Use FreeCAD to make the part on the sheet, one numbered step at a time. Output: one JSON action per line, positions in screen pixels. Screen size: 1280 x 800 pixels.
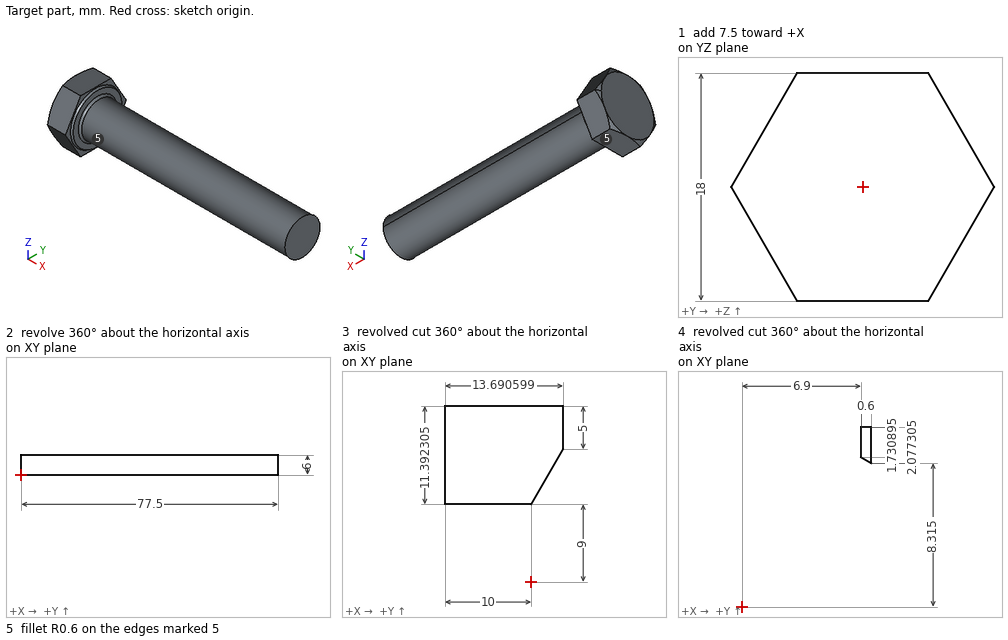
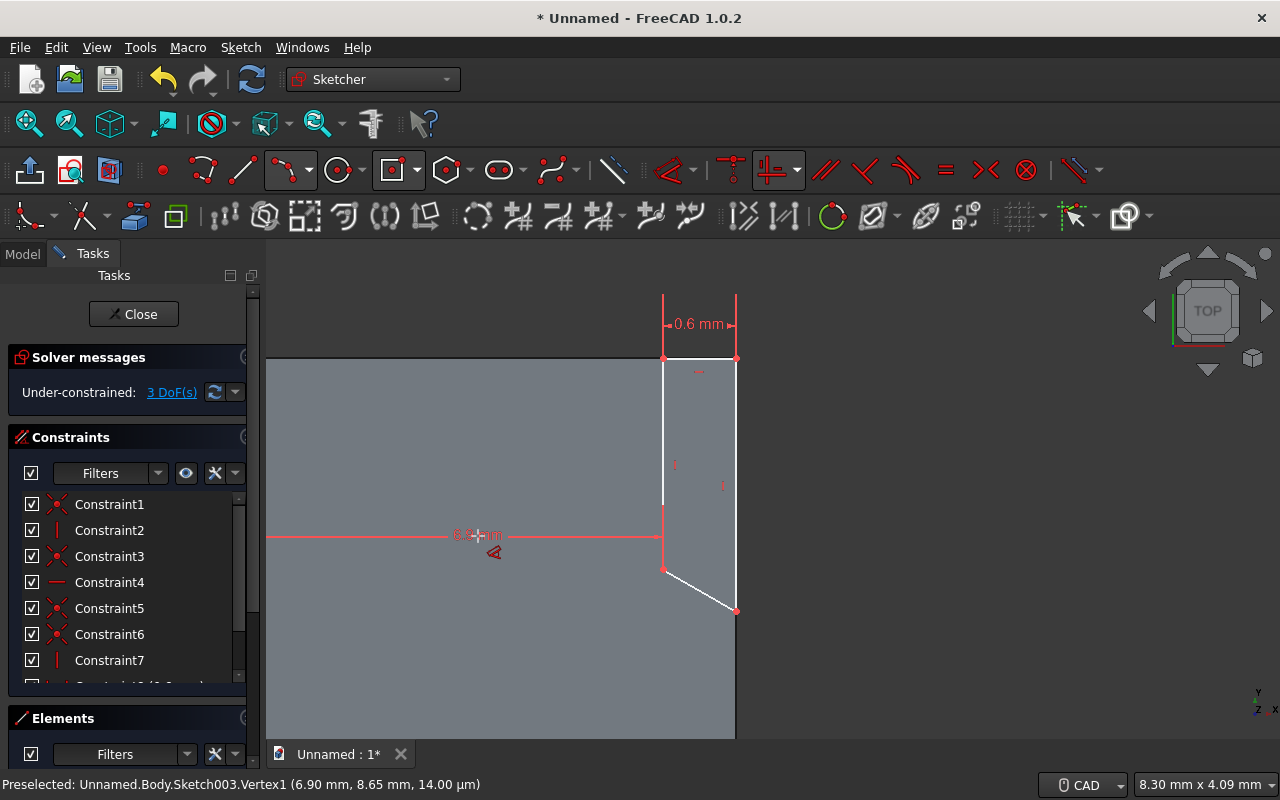
{"action": "left_click", "coordinate": [736, 612]}
{"action": "left_click", "coordinate": [770, 661]}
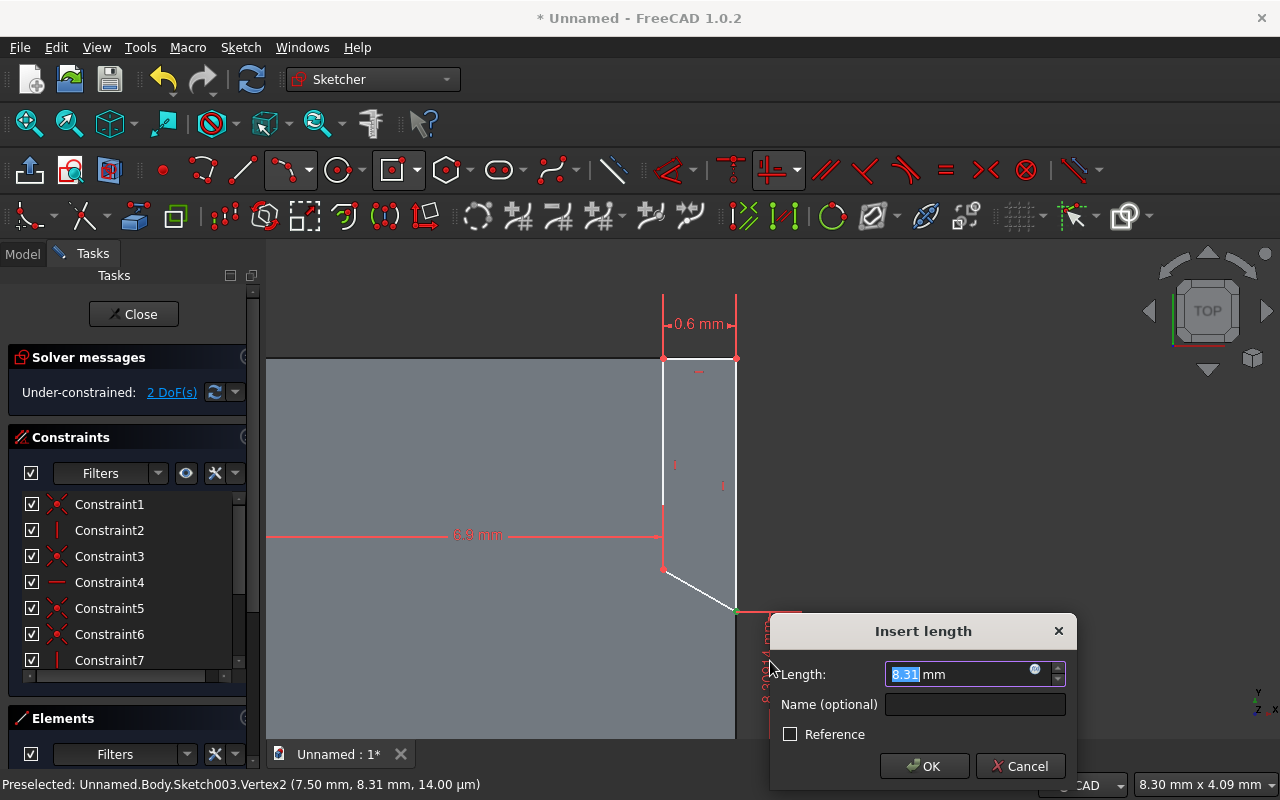
{"action": "type", "text": "8.315"}
{"action": "key", "text": "Return"}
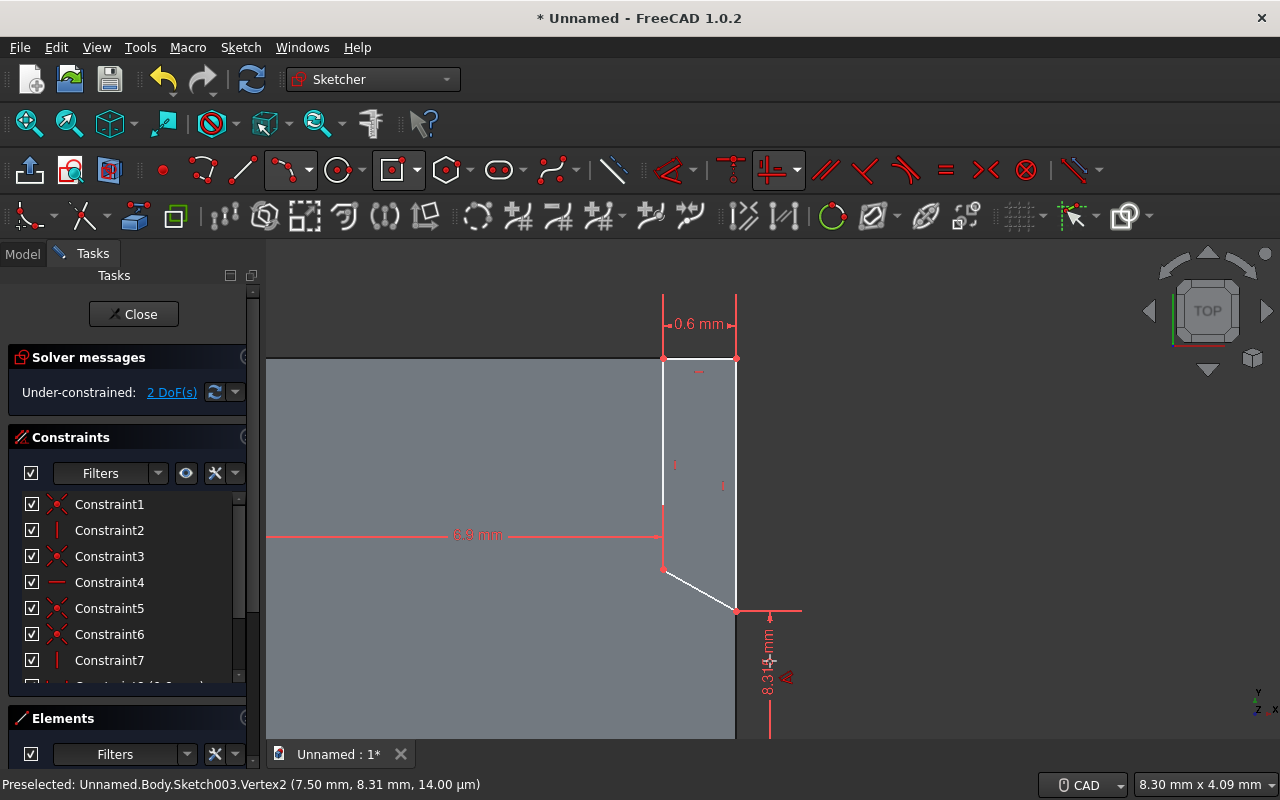
{"action": "left_click", "coordinate": [736, 536]}
{"action": "left_click", "coordinate": [770, 485]}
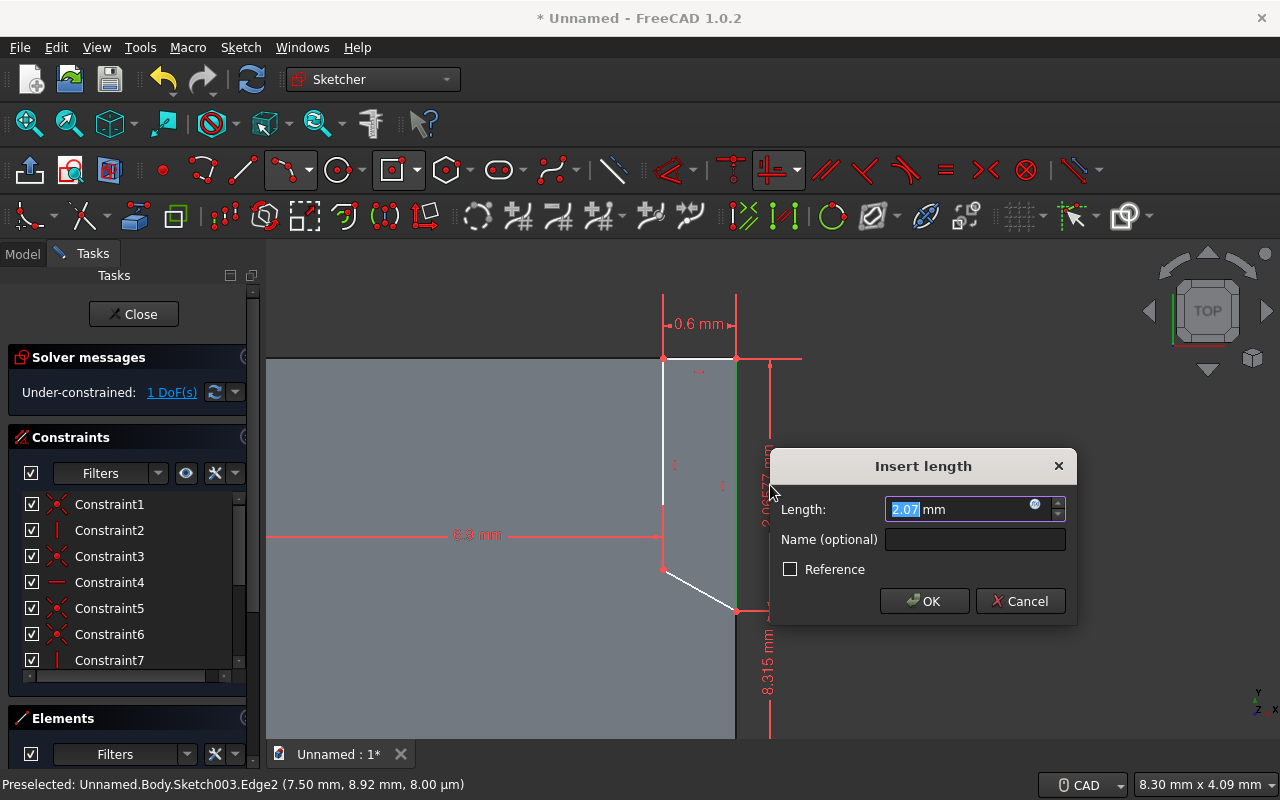
{"action": "type", "text": "2.077305"}
{"action": "key", "text": "Return"}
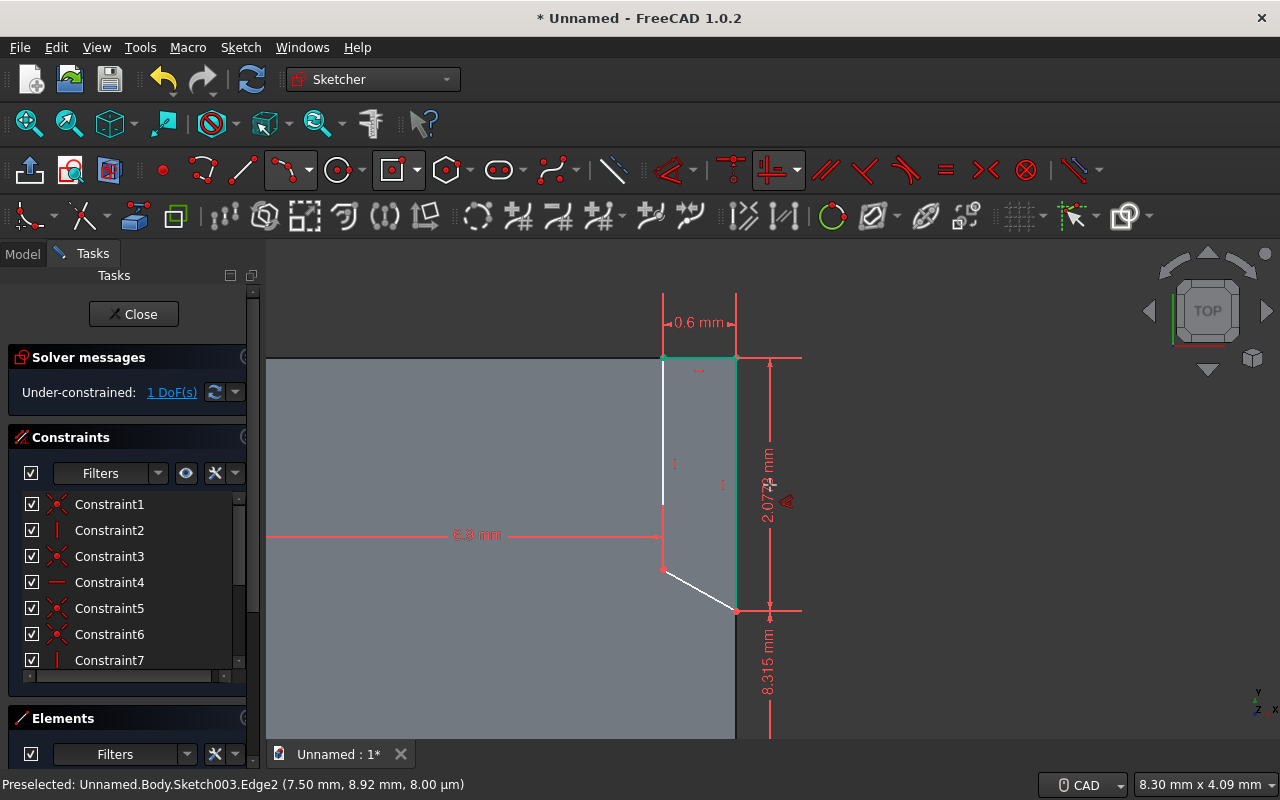
{"action": "left_click", "coordinate": [663, 421]}
{"action": "left_click", "coordinate": [629, 464]}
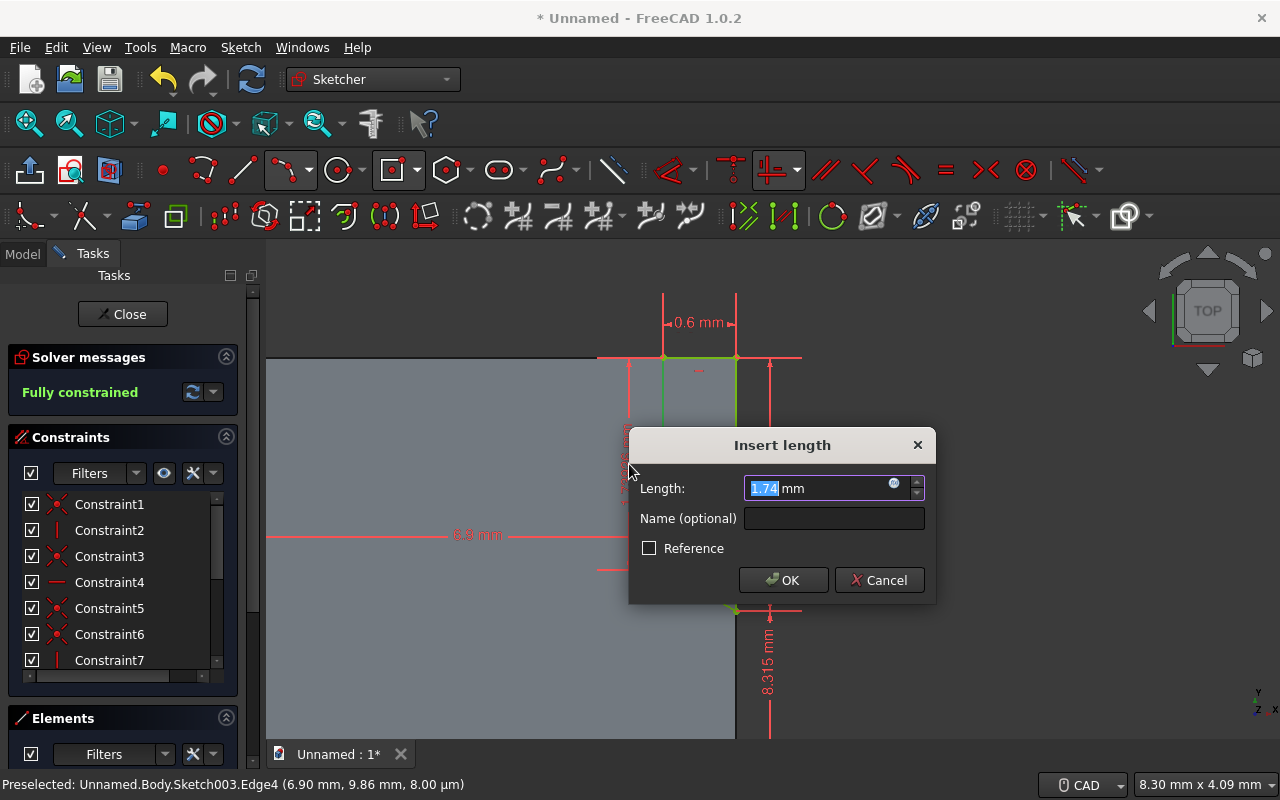
{"action": "type", "text": "1.730895"}
{"action": "key", "text": "Return"}
{"action": "key", "text": "Escape"}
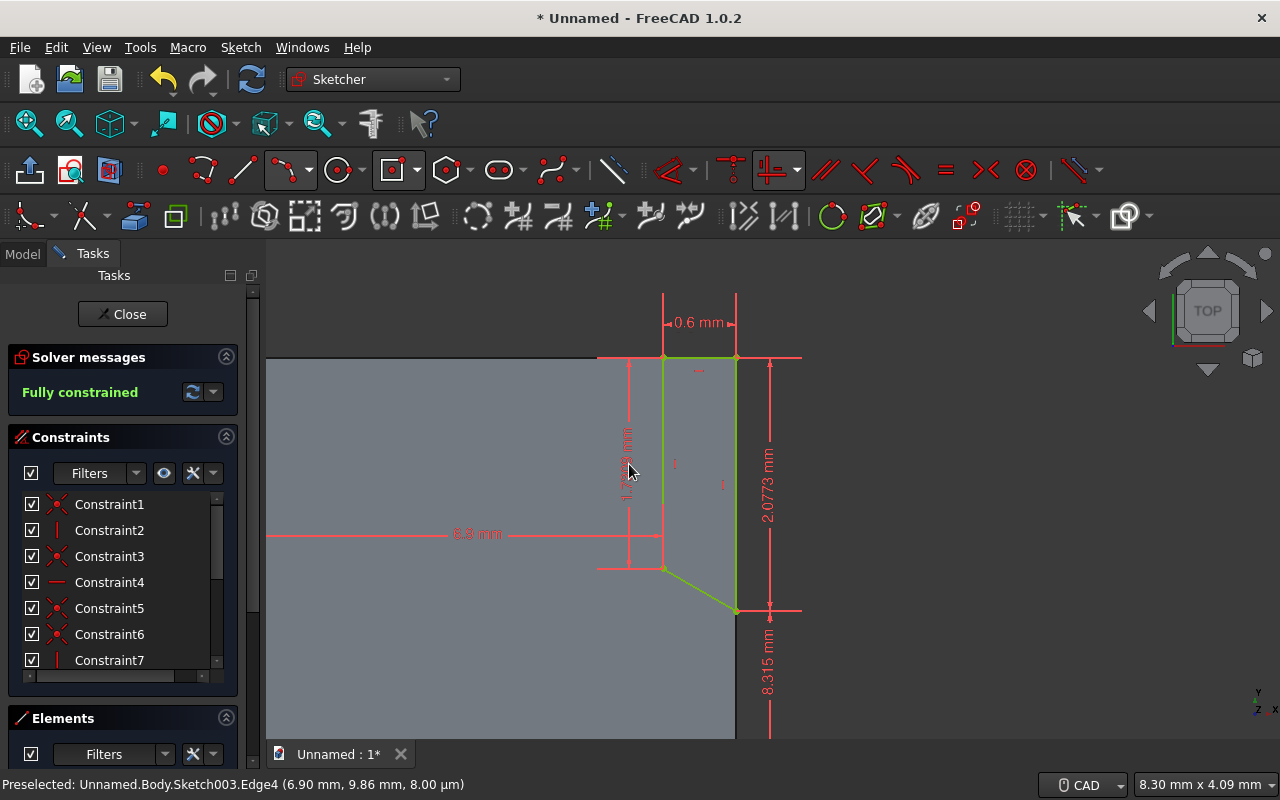
{"action": "left_click", "coordinate": [123, 314]}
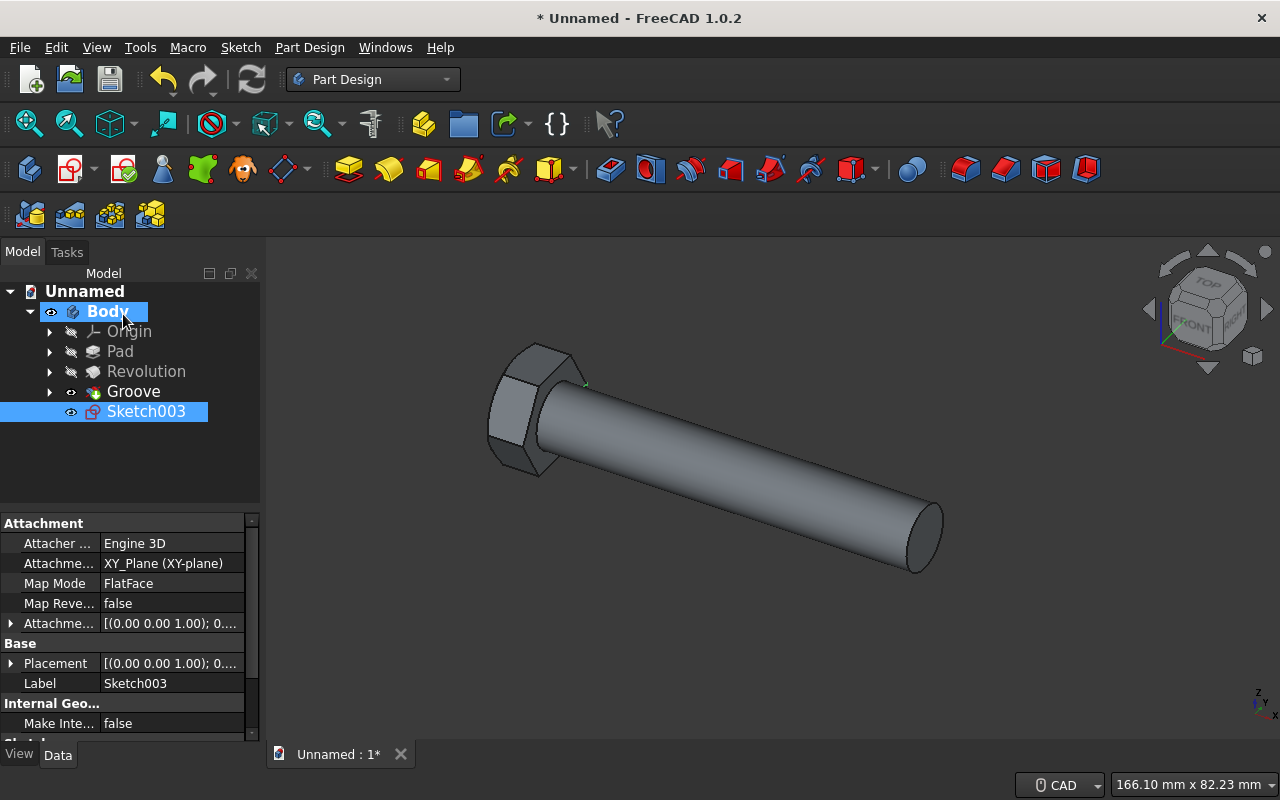
{"action": "left_click", "coordinate": [692, 170]}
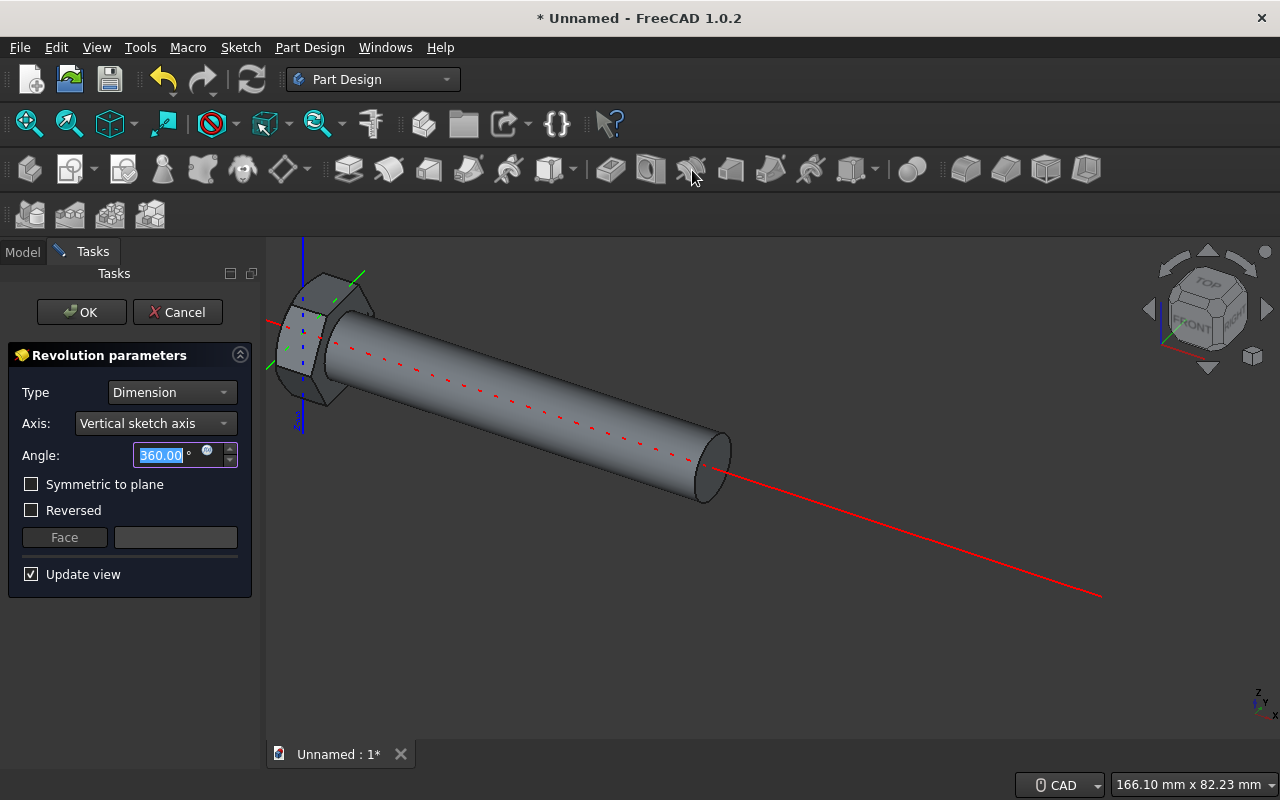
{"action": "left_click", "coordinate": [156, 424]}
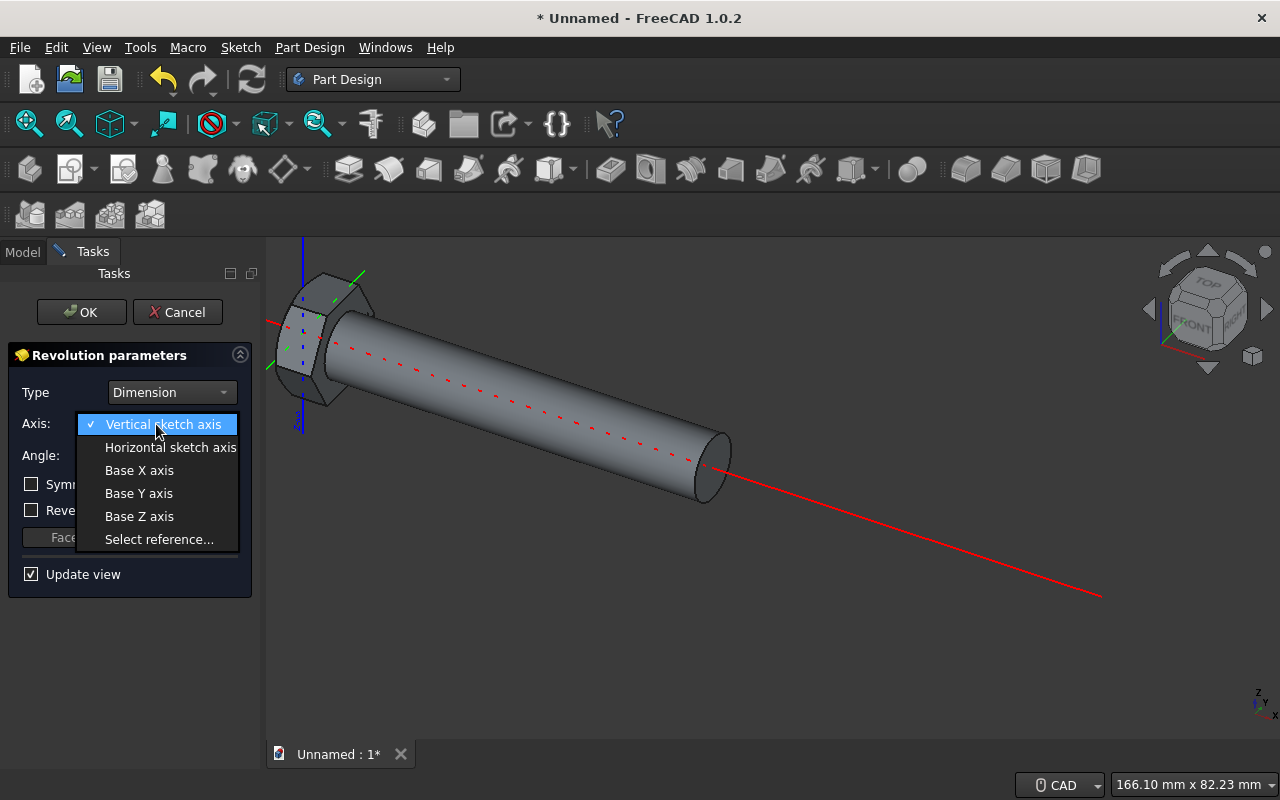
{"action": "left_click", "coordinate": [156, 448]}